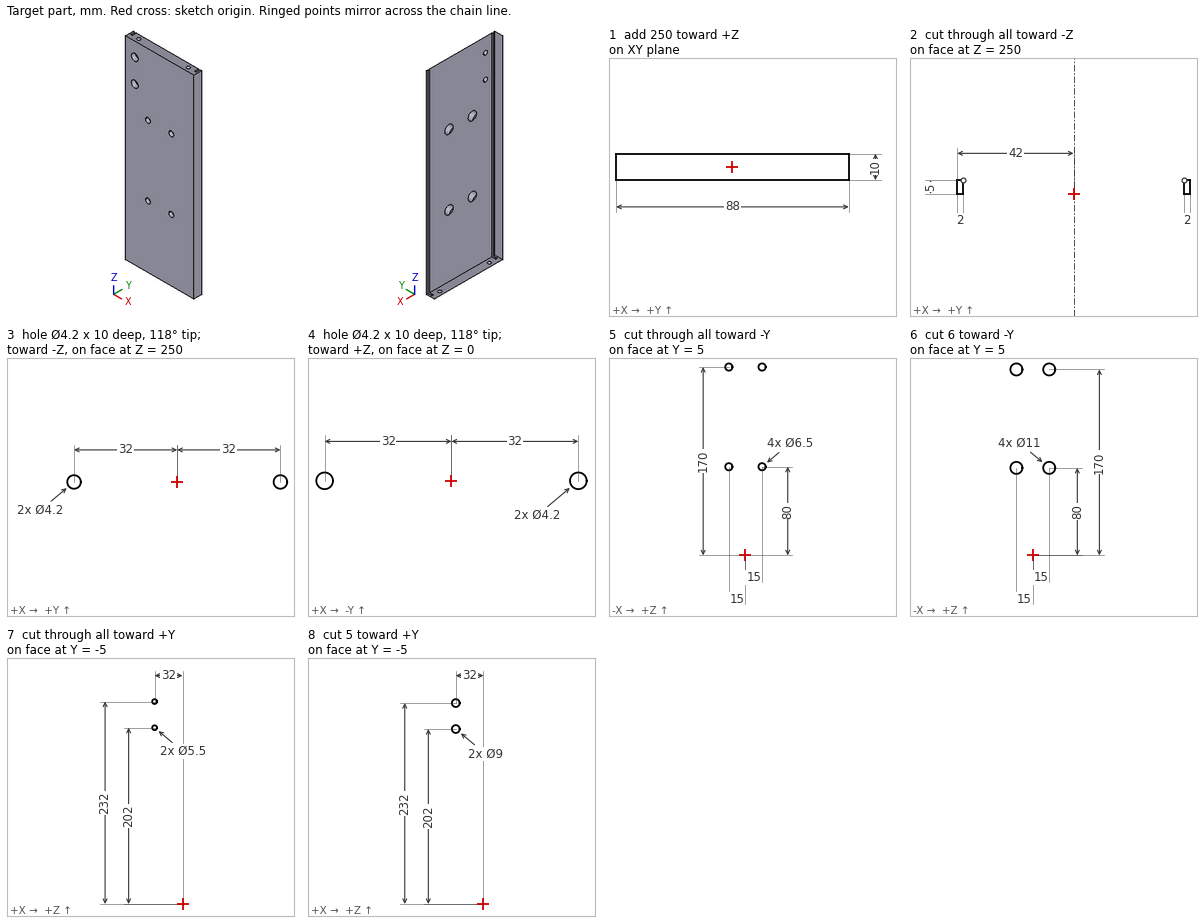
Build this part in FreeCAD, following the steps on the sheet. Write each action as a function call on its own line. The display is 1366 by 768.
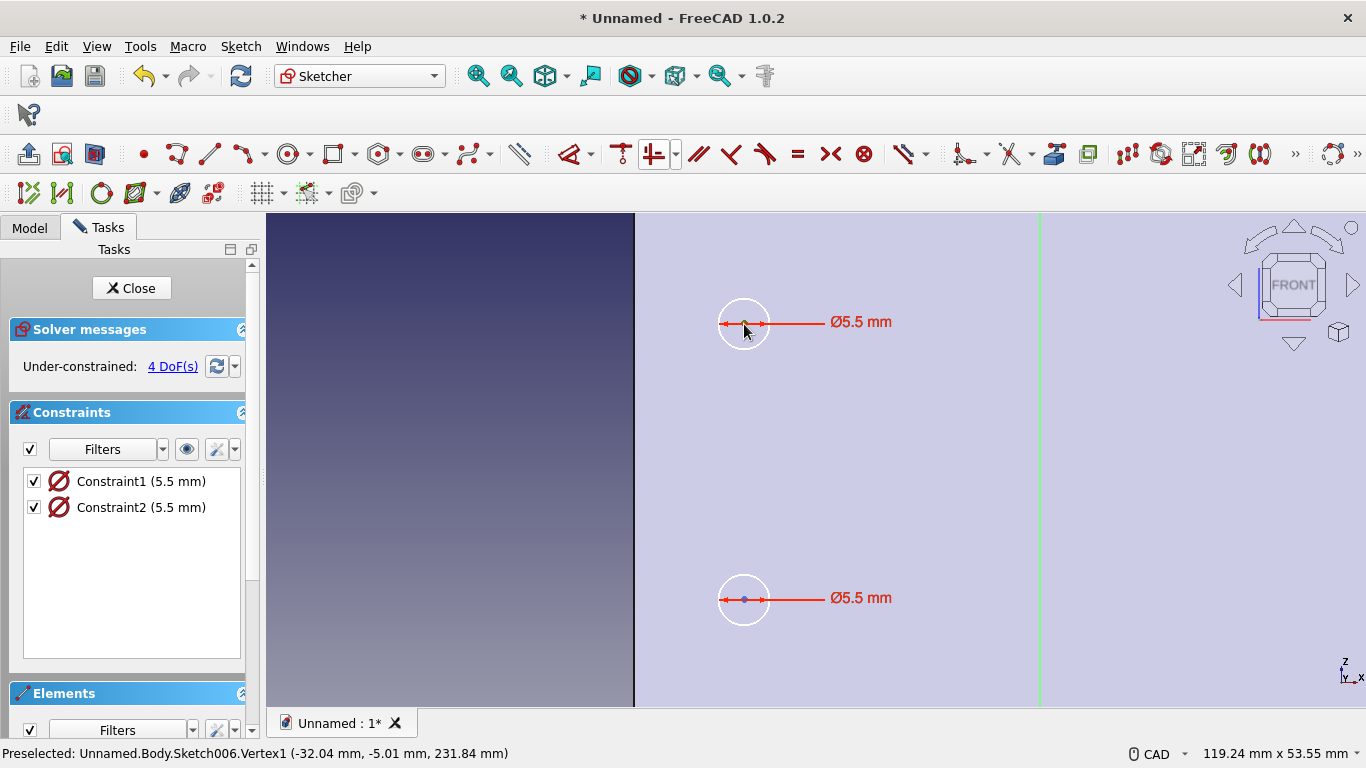
click(744, 600)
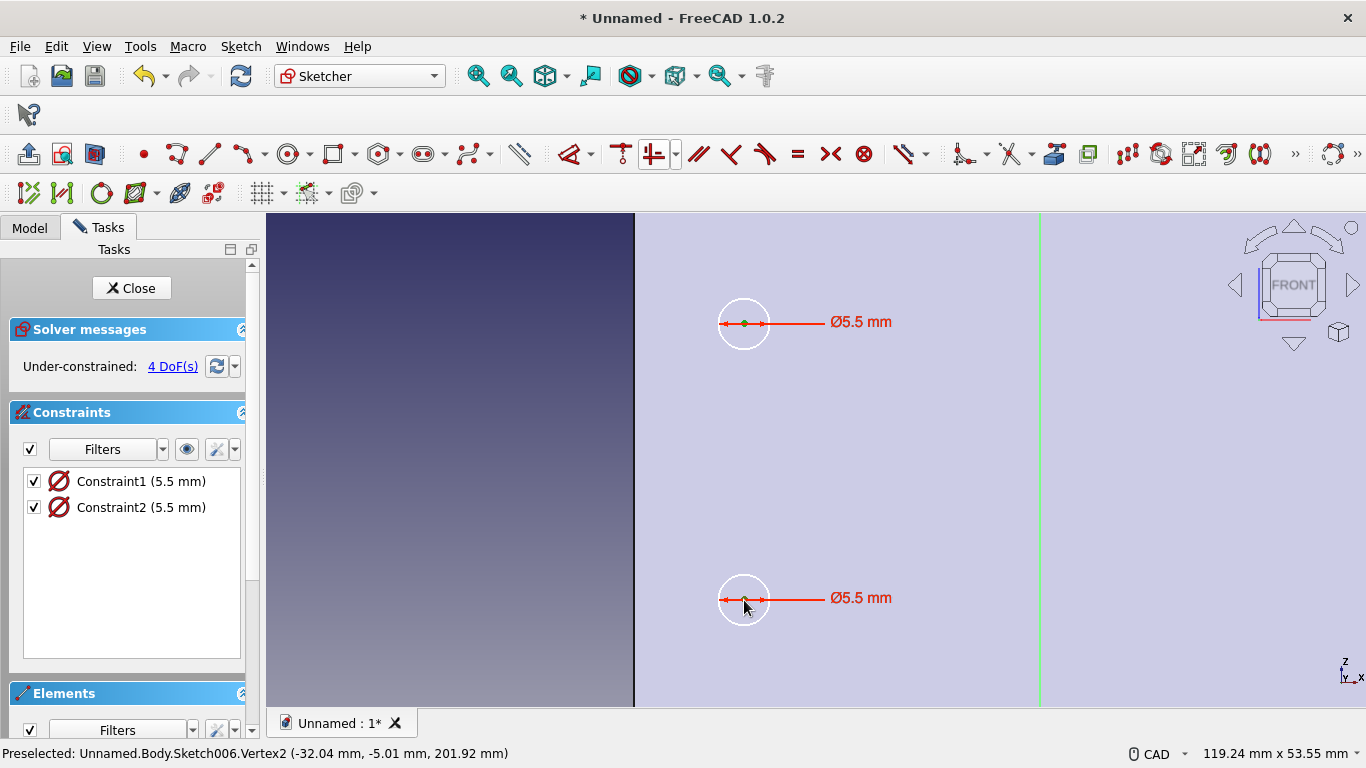
key(v)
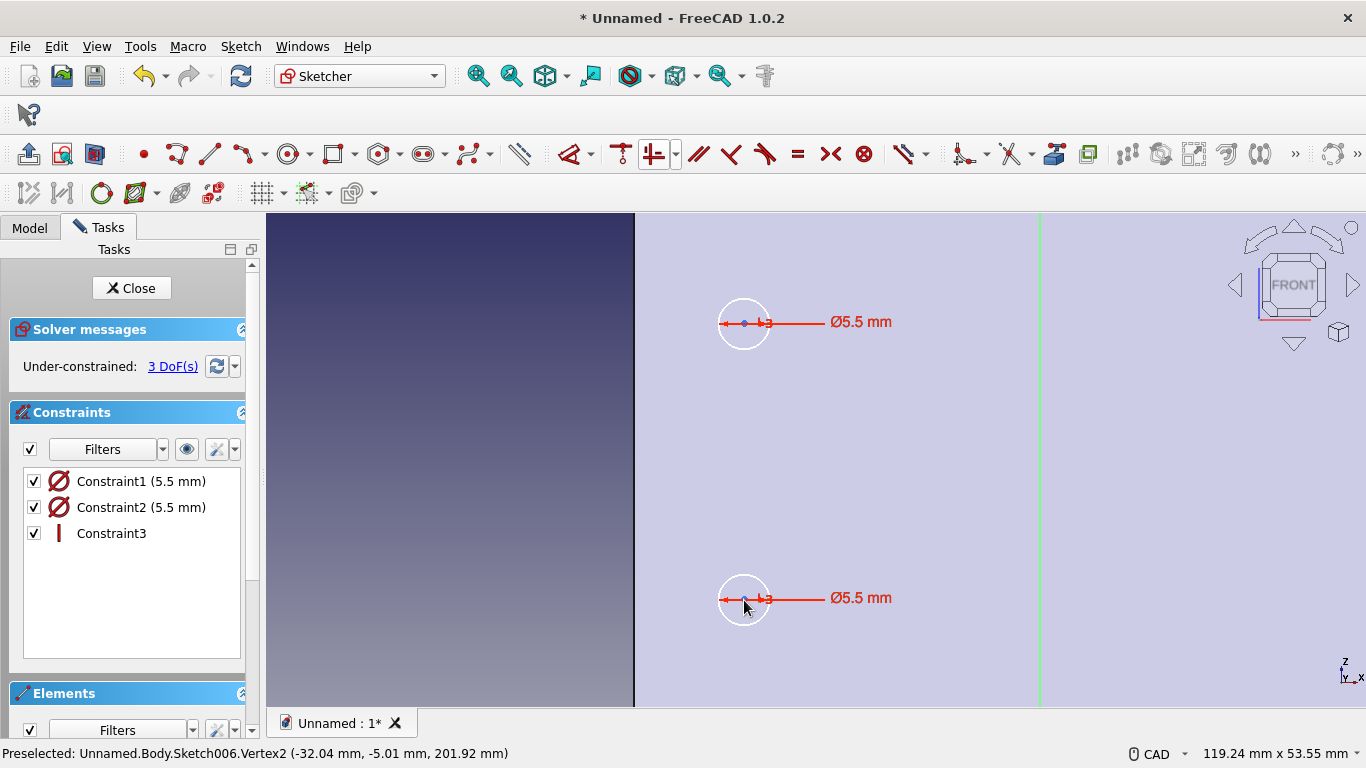
click(568, 154)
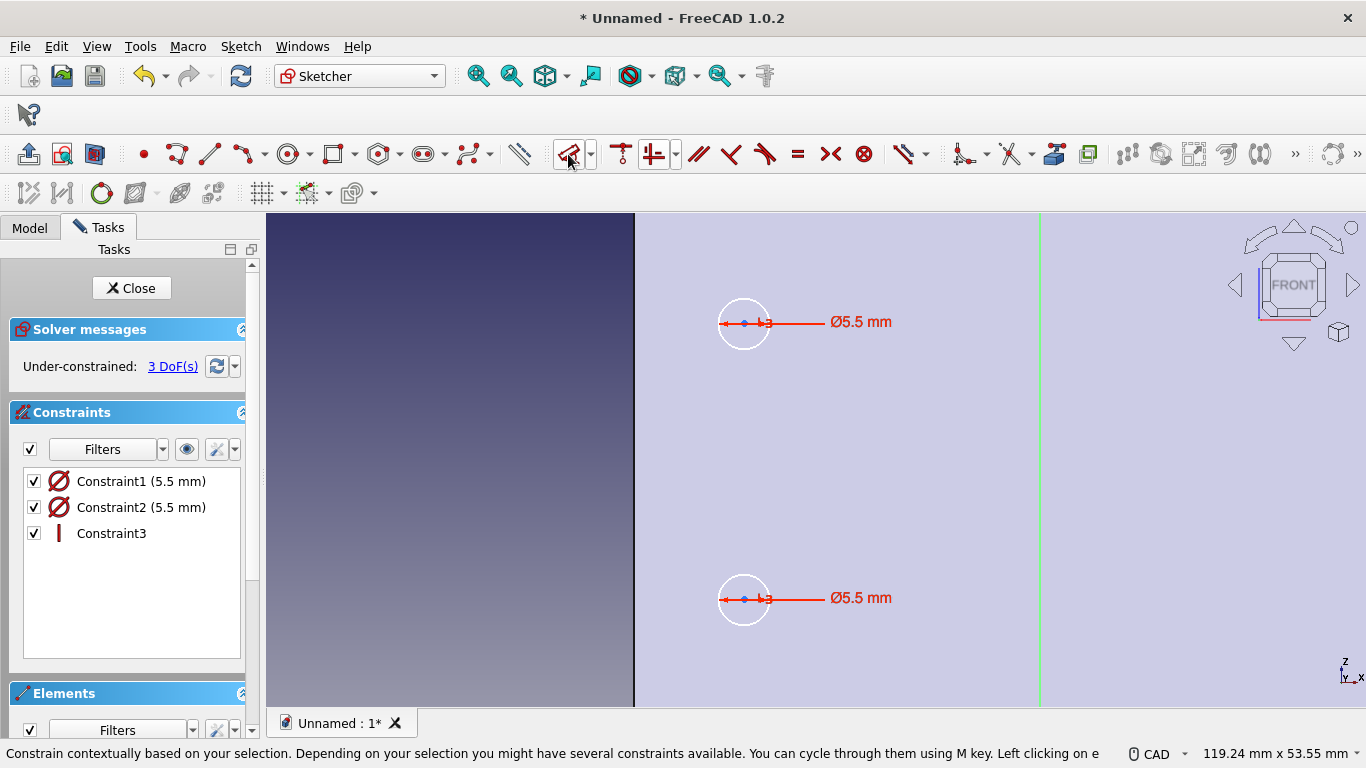
click(744, 324)
click(892, 290)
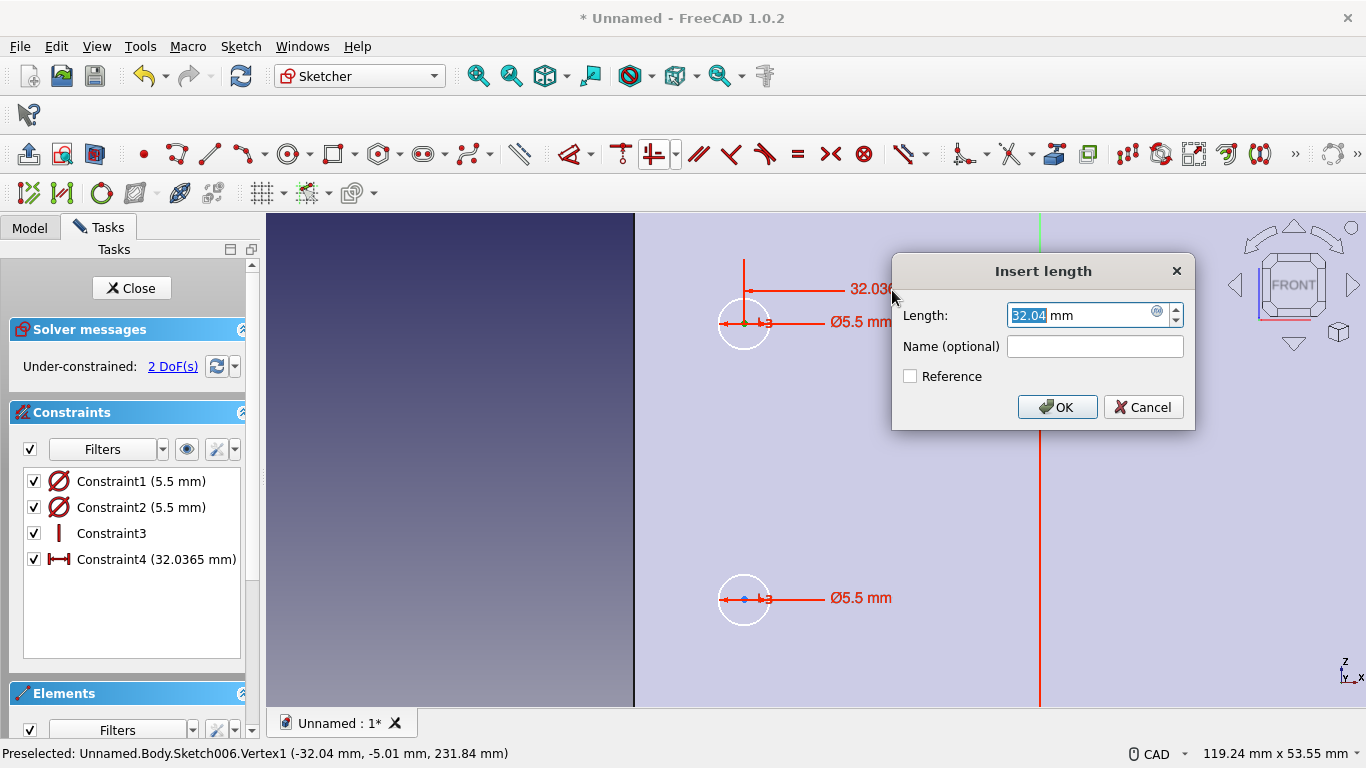
text(32)
key(Return)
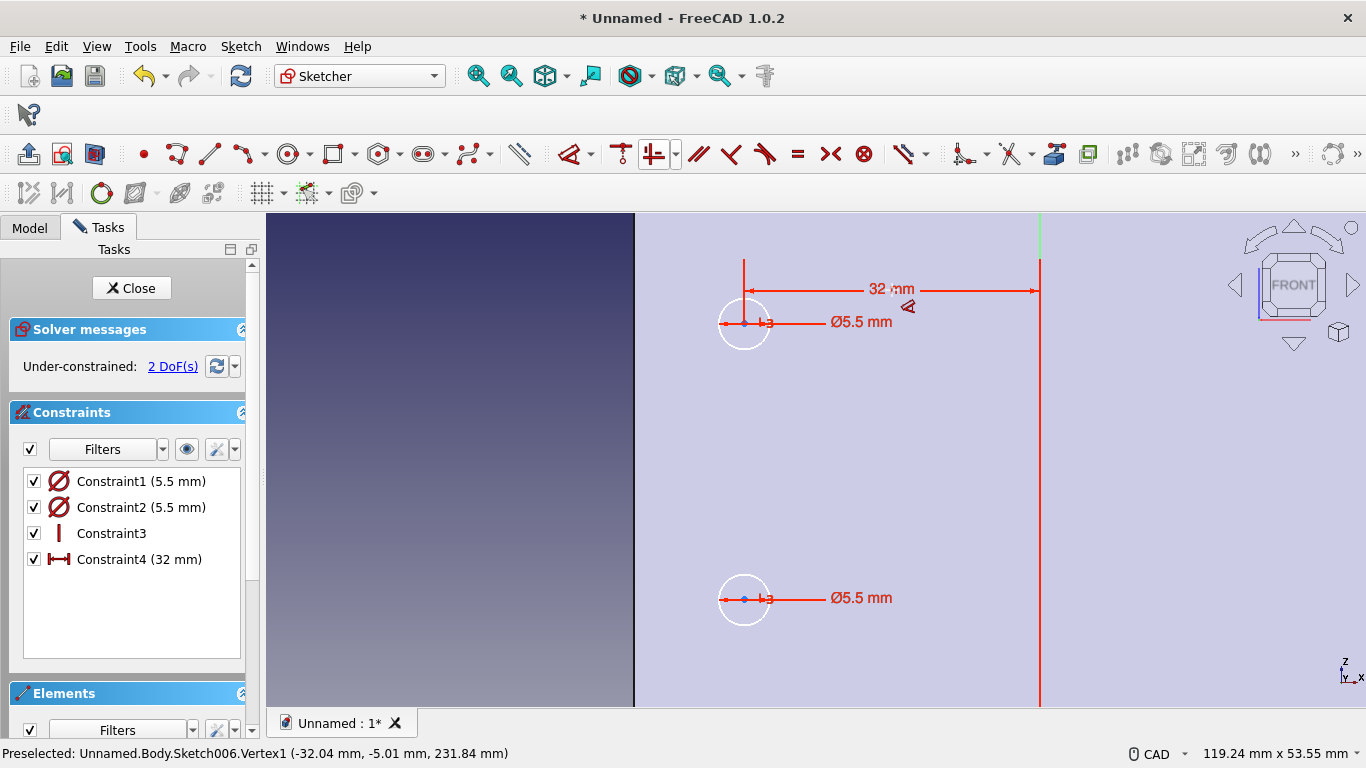
click(744, 324)
click(1074, 502)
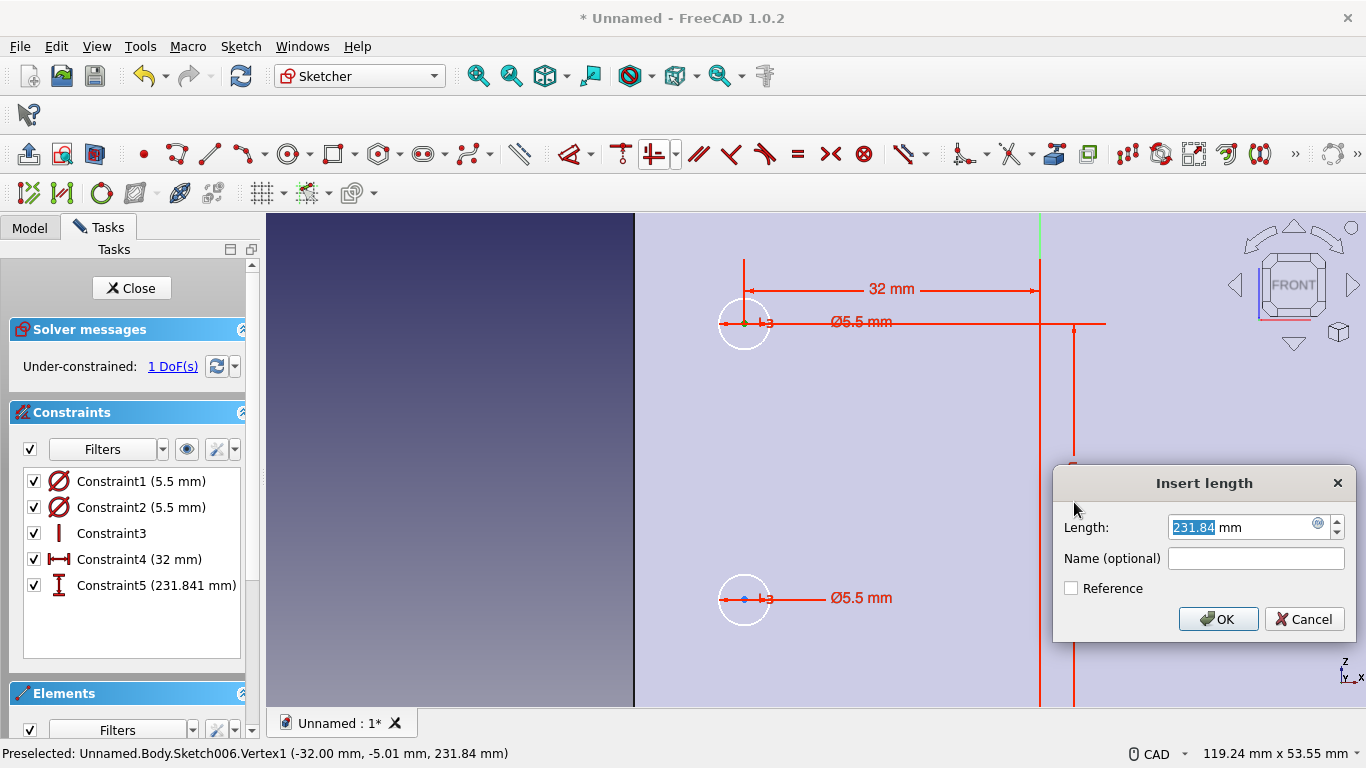
text(232)
key(Return)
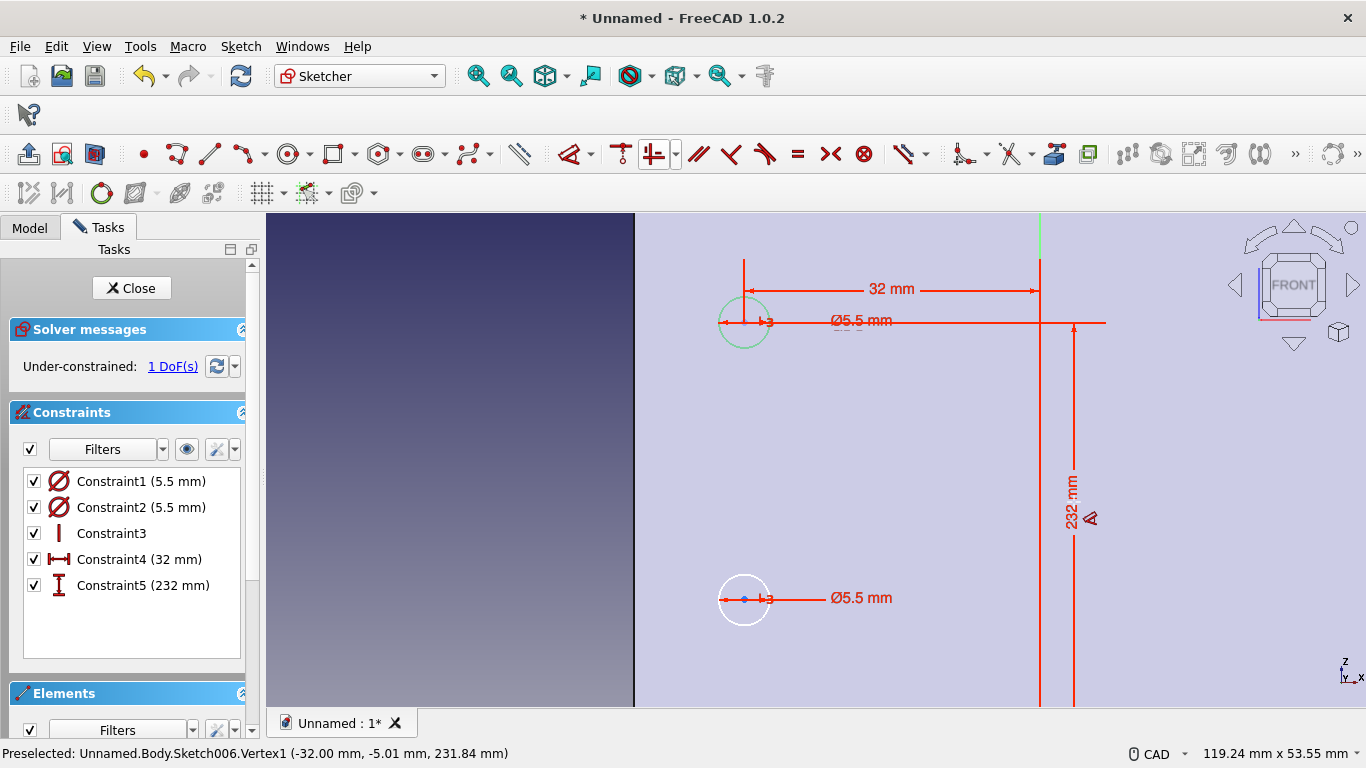
click(744, 600)
click(1074, 640)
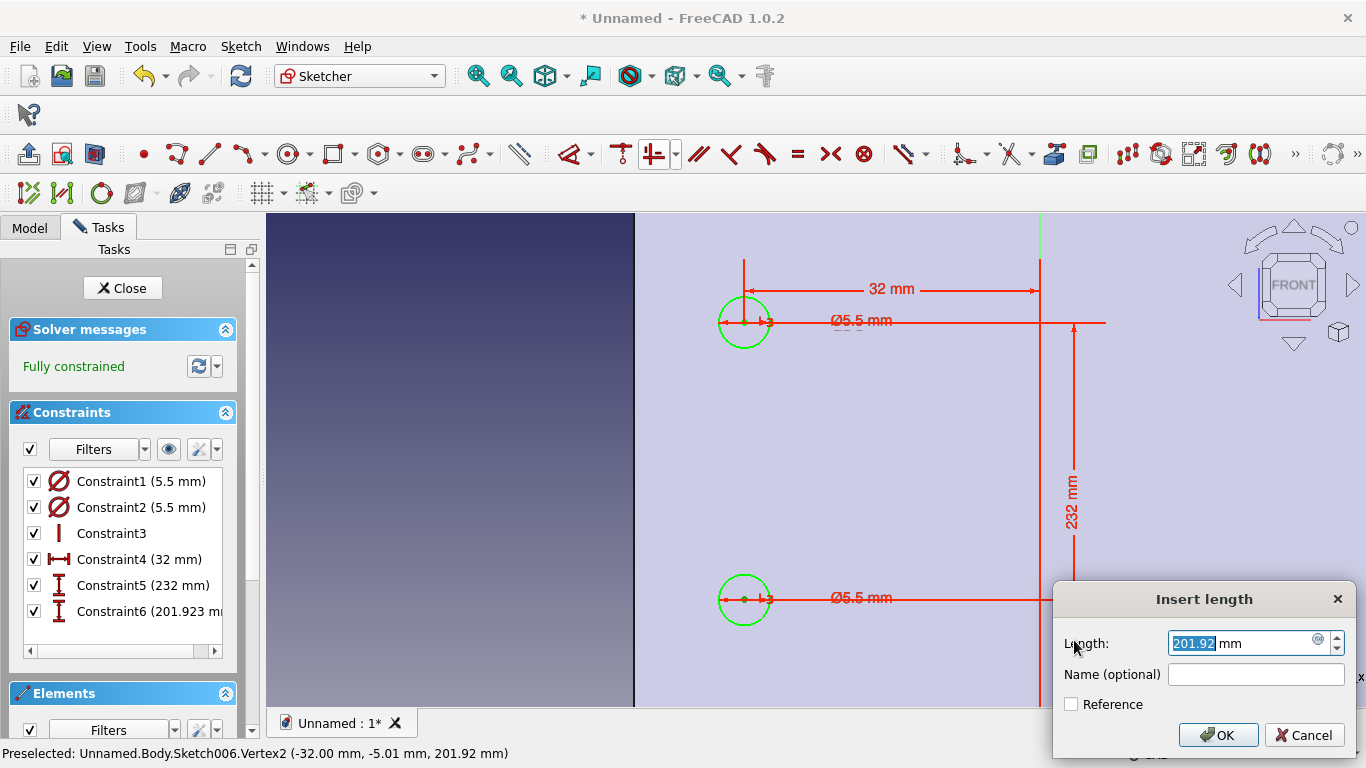
text(202)
key(Return)
key(Escape)